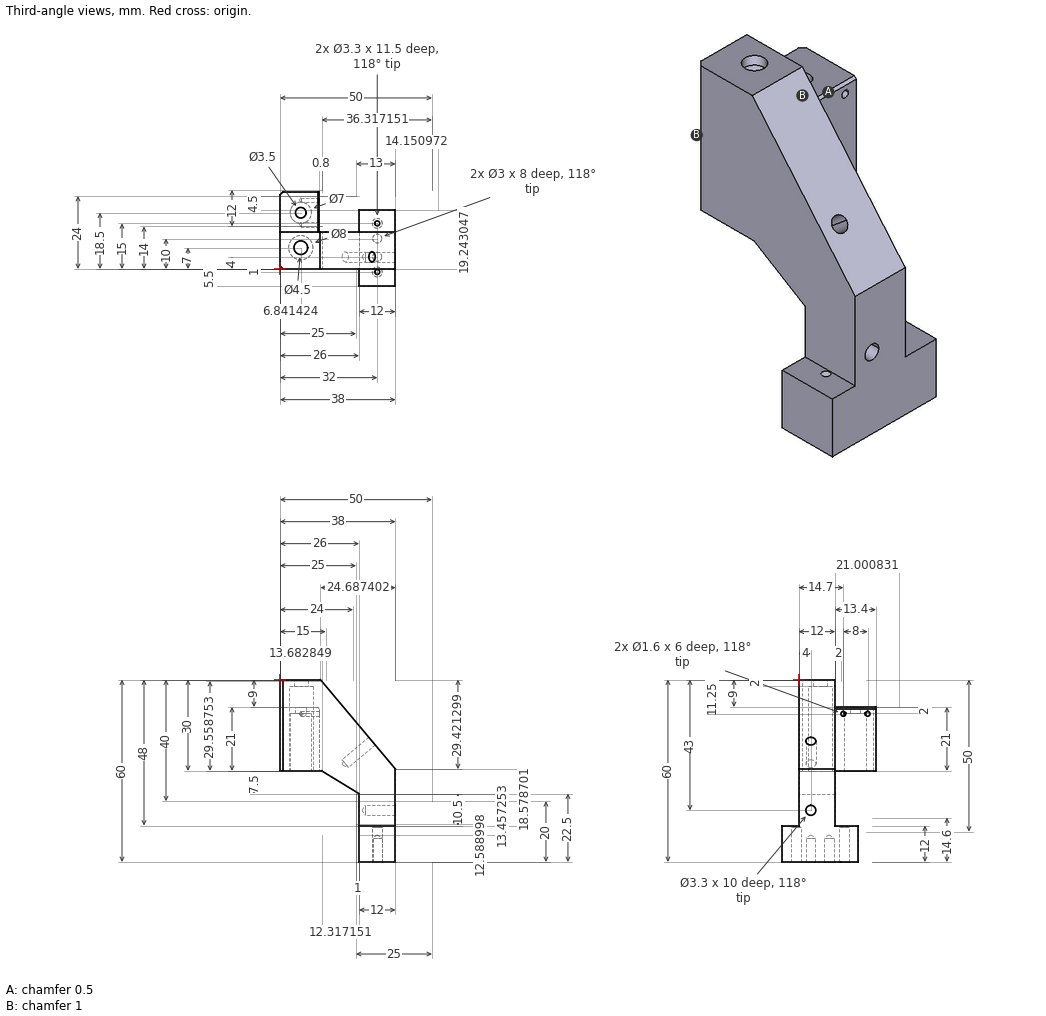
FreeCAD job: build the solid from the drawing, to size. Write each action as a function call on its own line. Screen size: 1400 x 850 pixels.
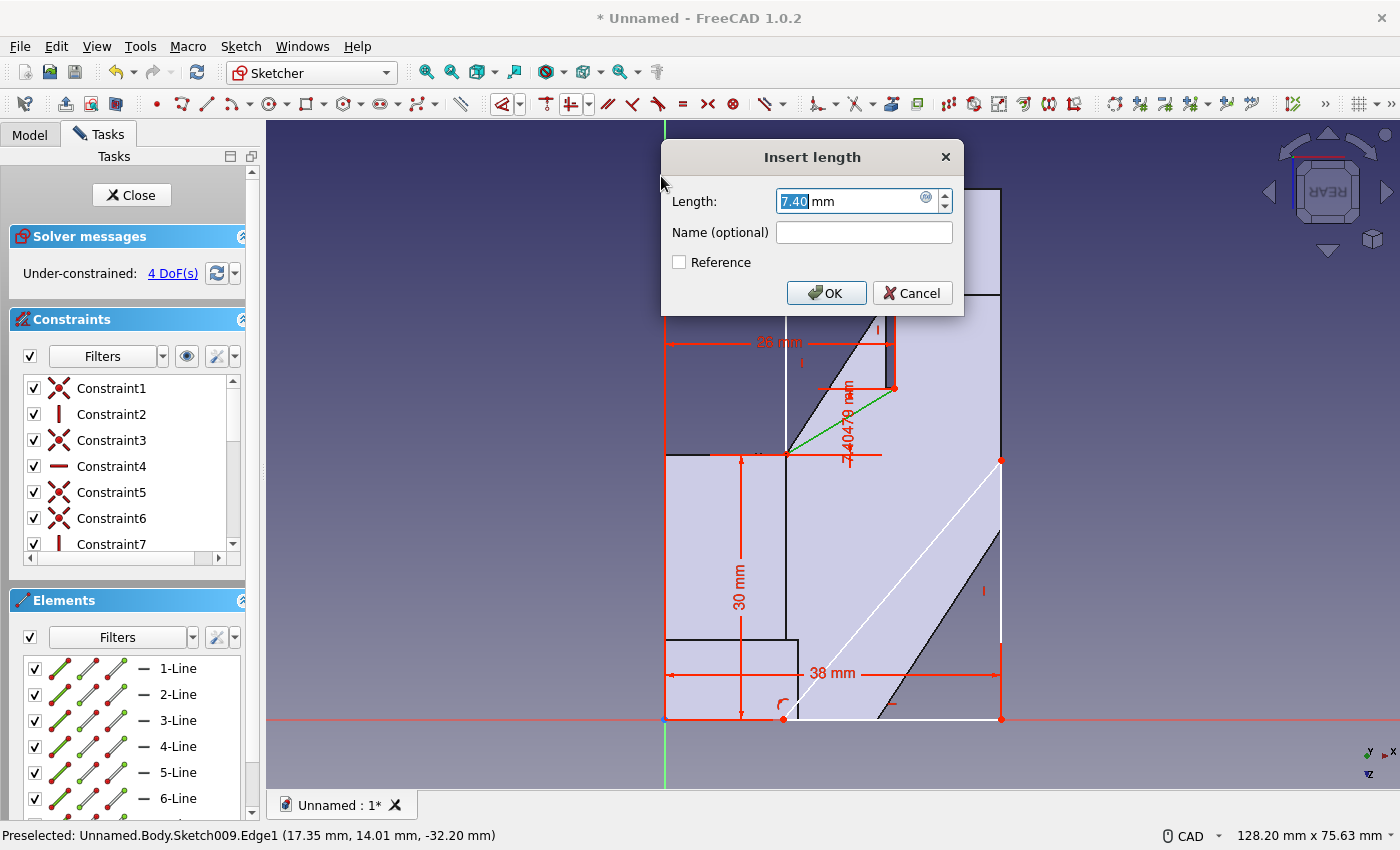
text(7.5)
key(Return)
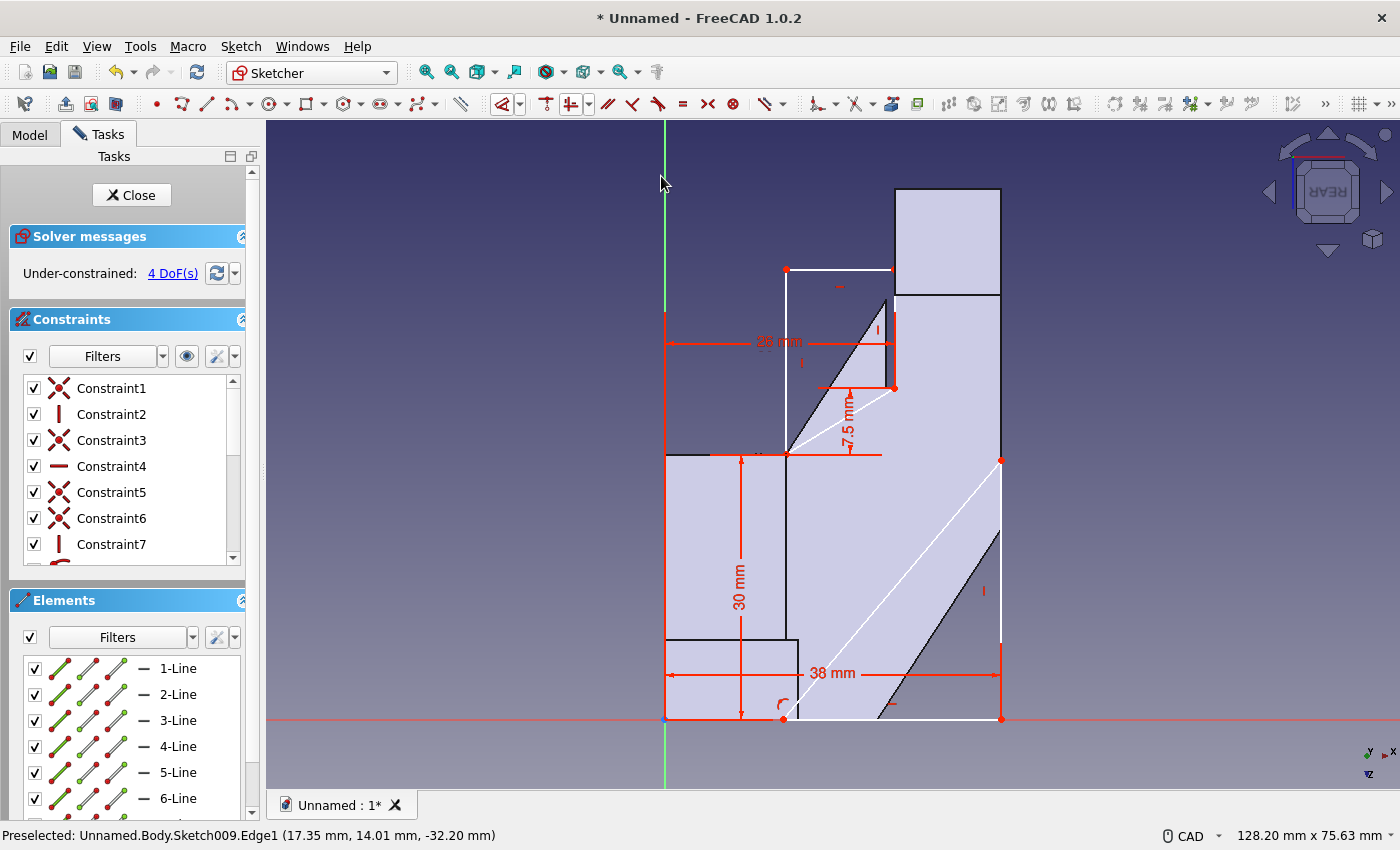
click(895, 353)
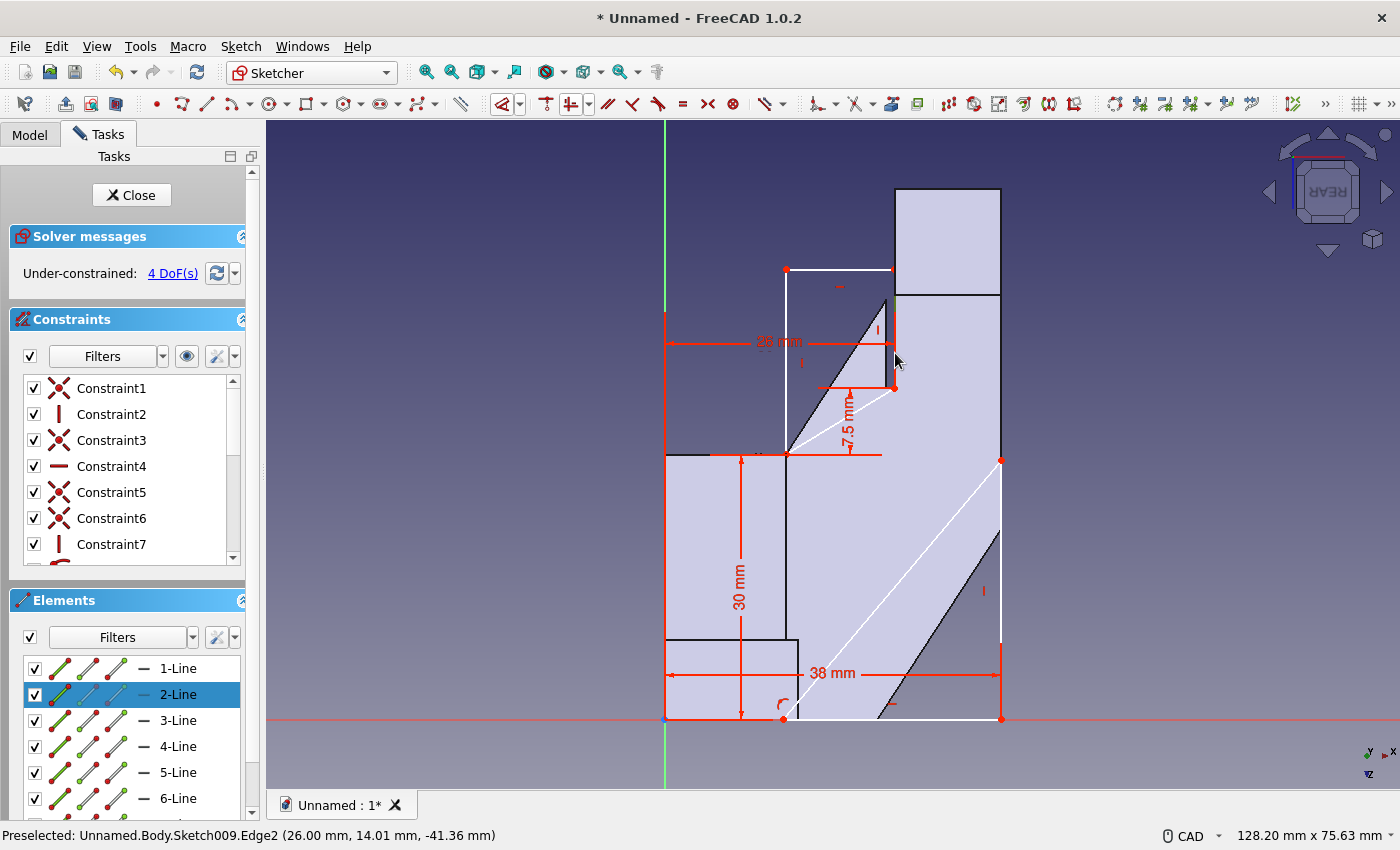
click(520, 104)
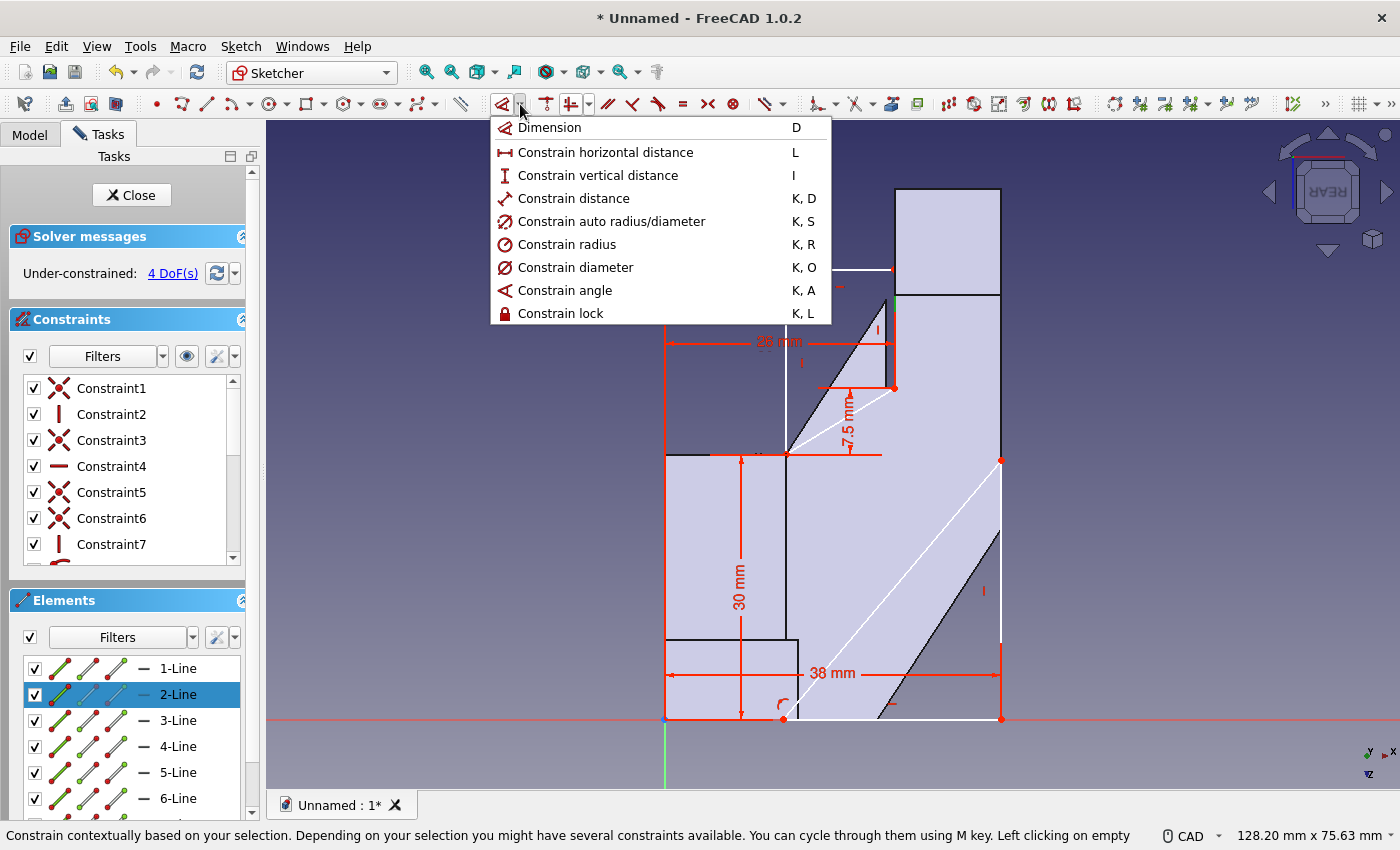
click(661, 176)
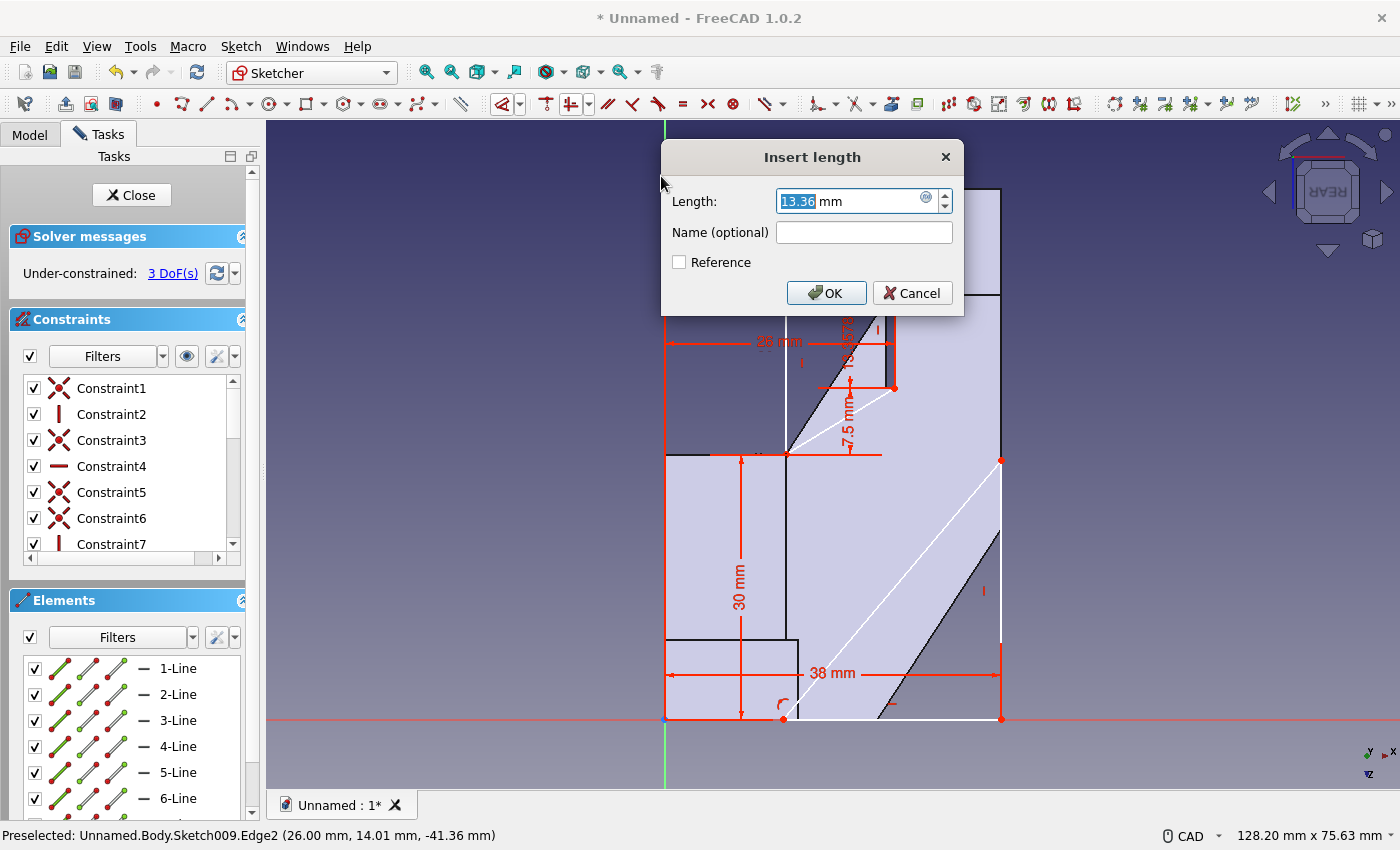
text(13.457253)
key(Return)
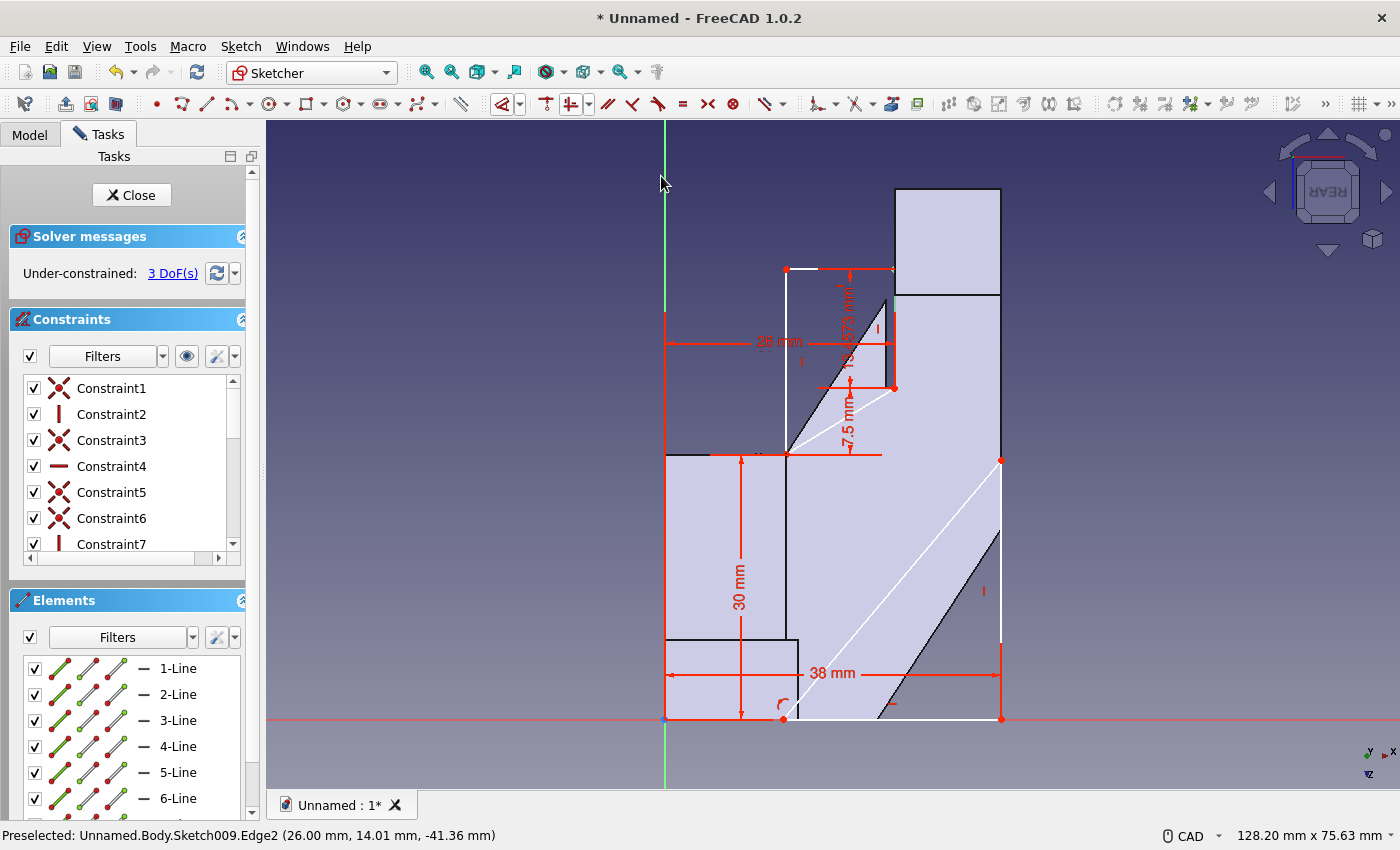
click(862, 269)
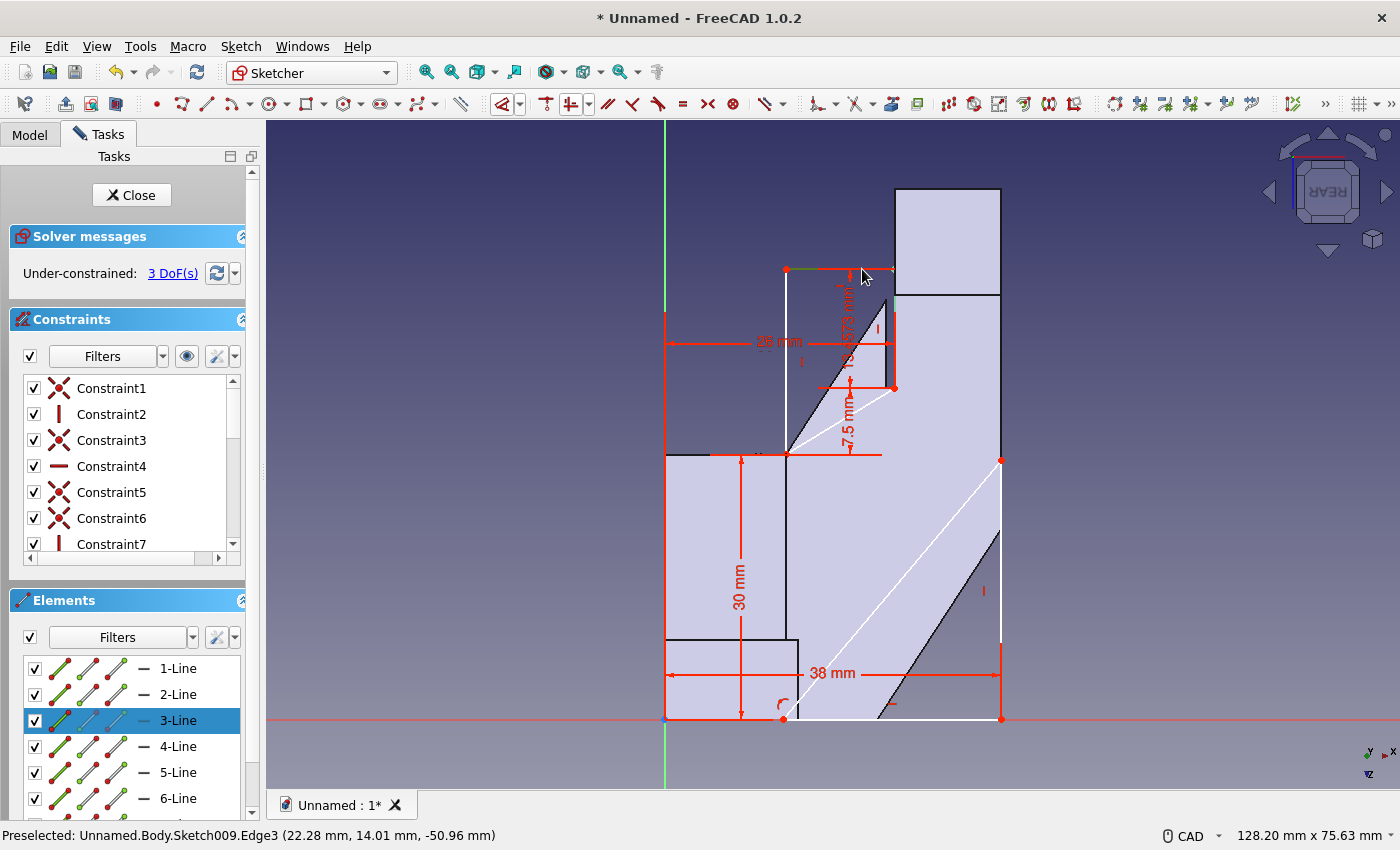
click(520, 104)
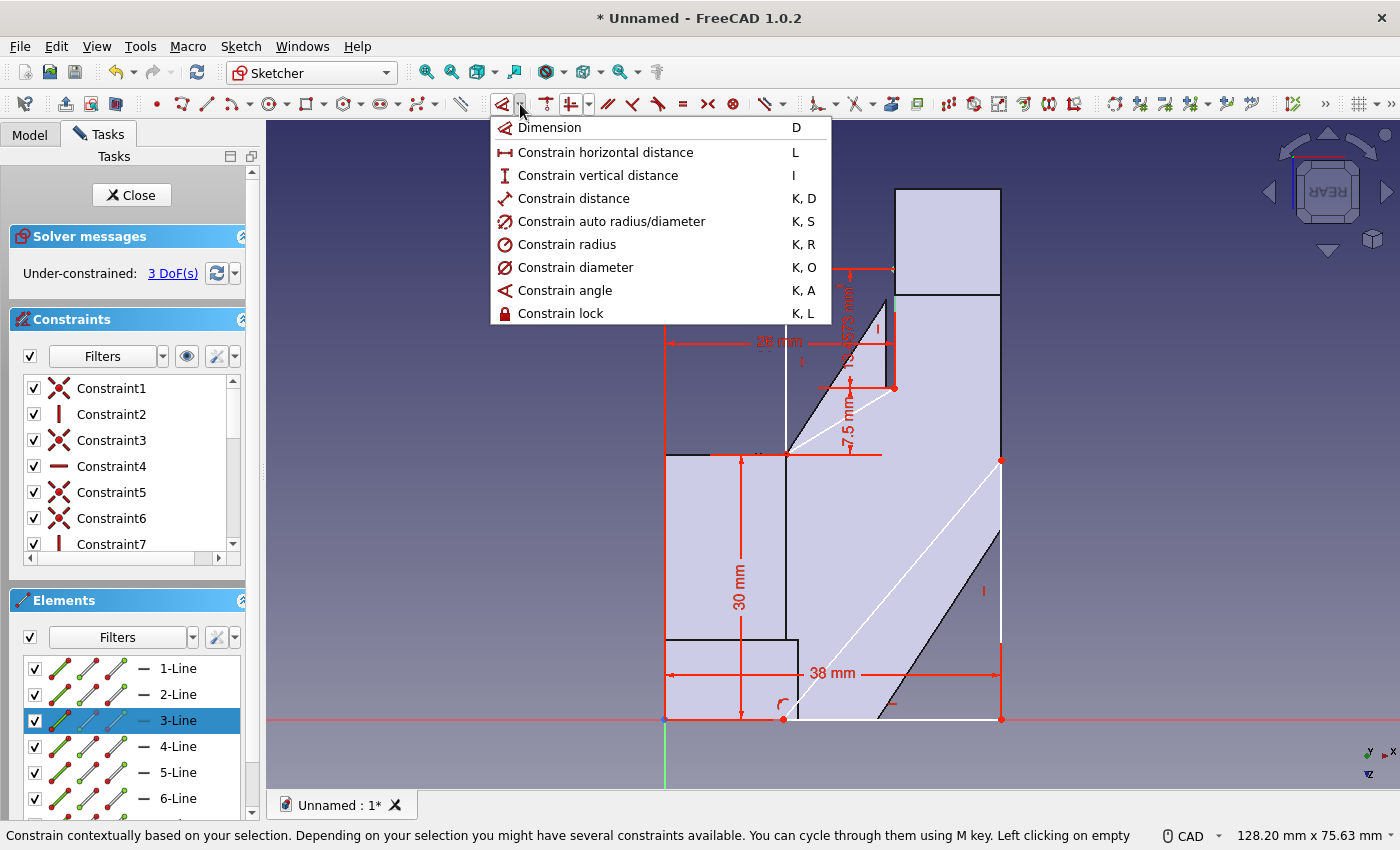
click(661, 152)